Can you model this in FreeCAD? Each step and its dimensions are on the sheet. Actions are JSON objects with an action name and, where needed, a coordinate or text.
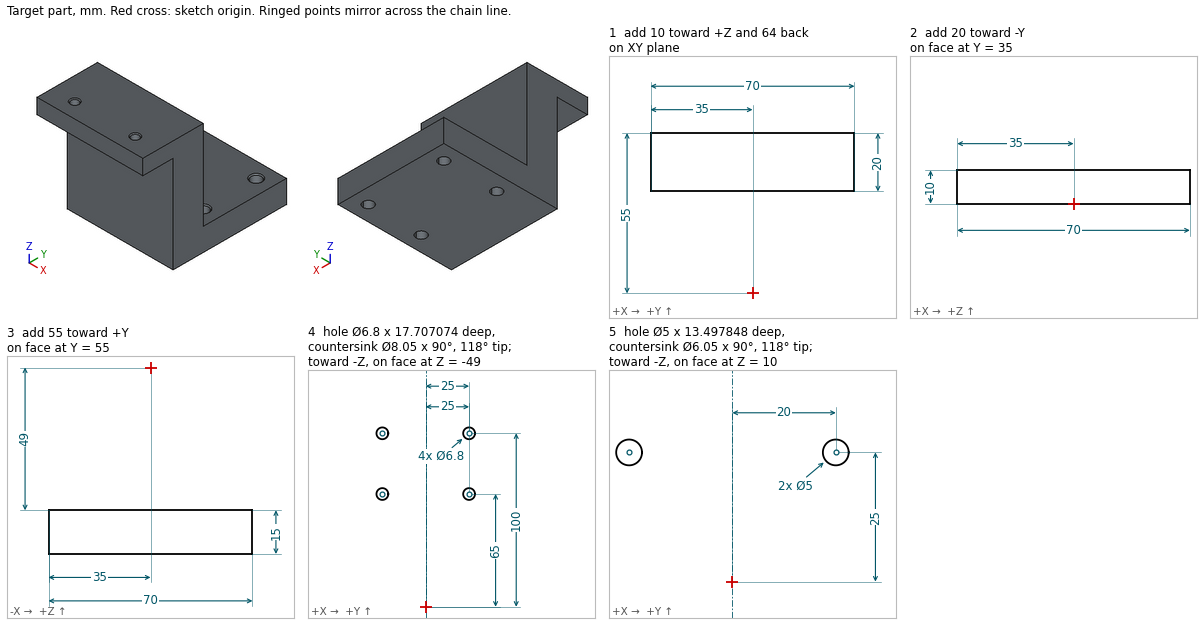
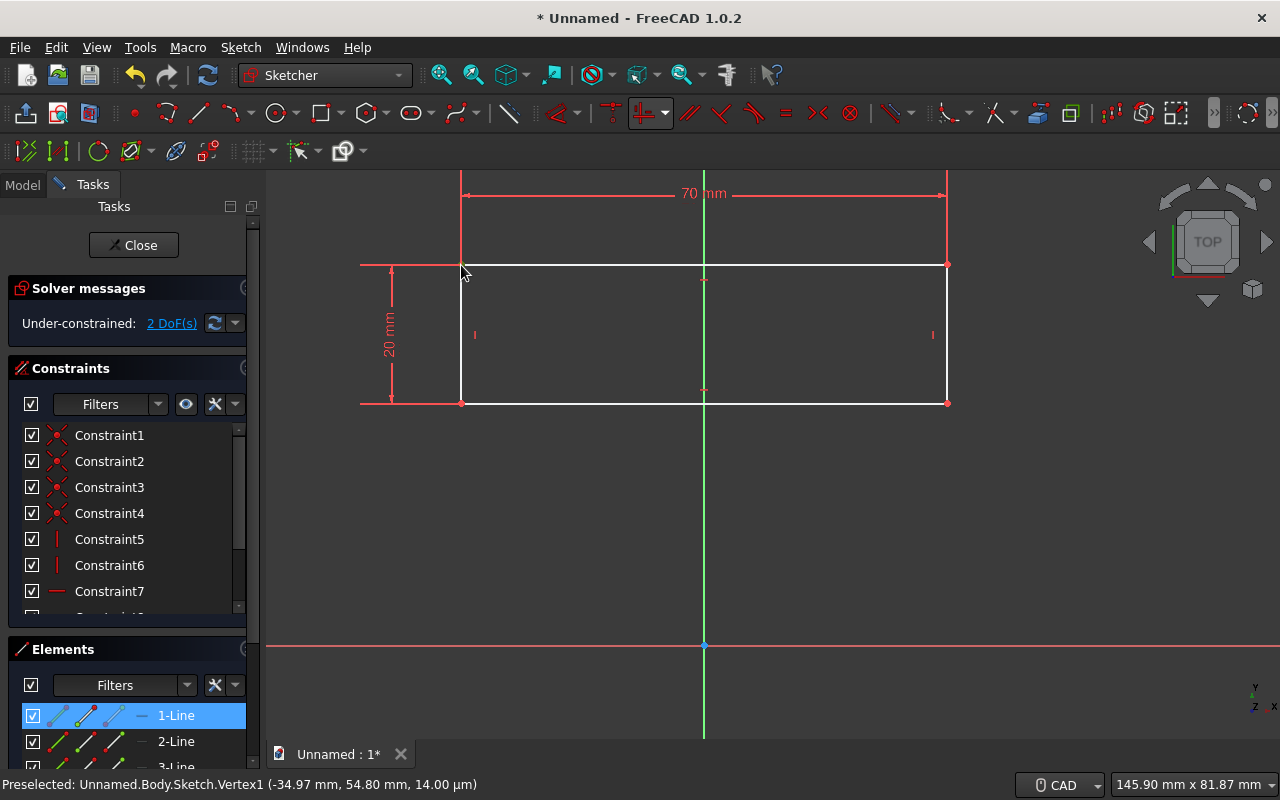
{"action": "left_click", "coordinate": [580, 114]}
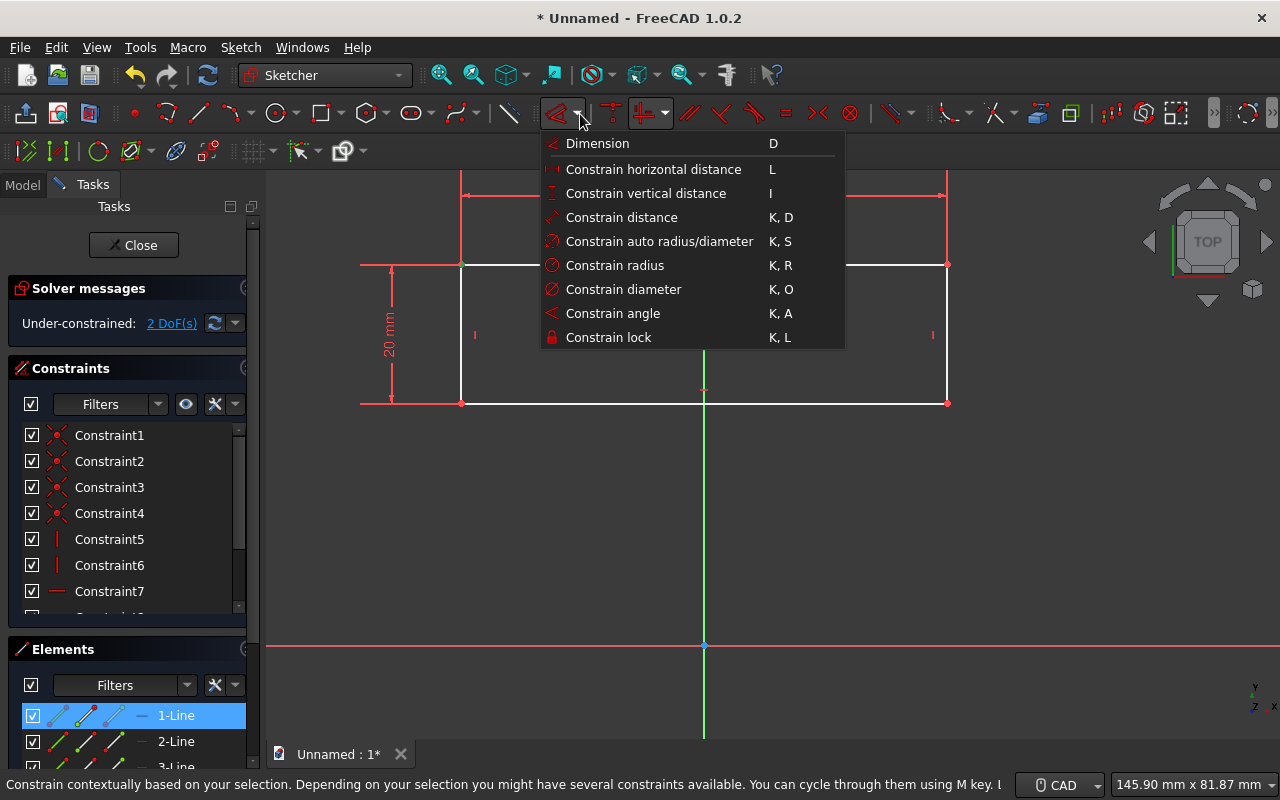
{"action": "left_click", "coordinate": [693, 169]}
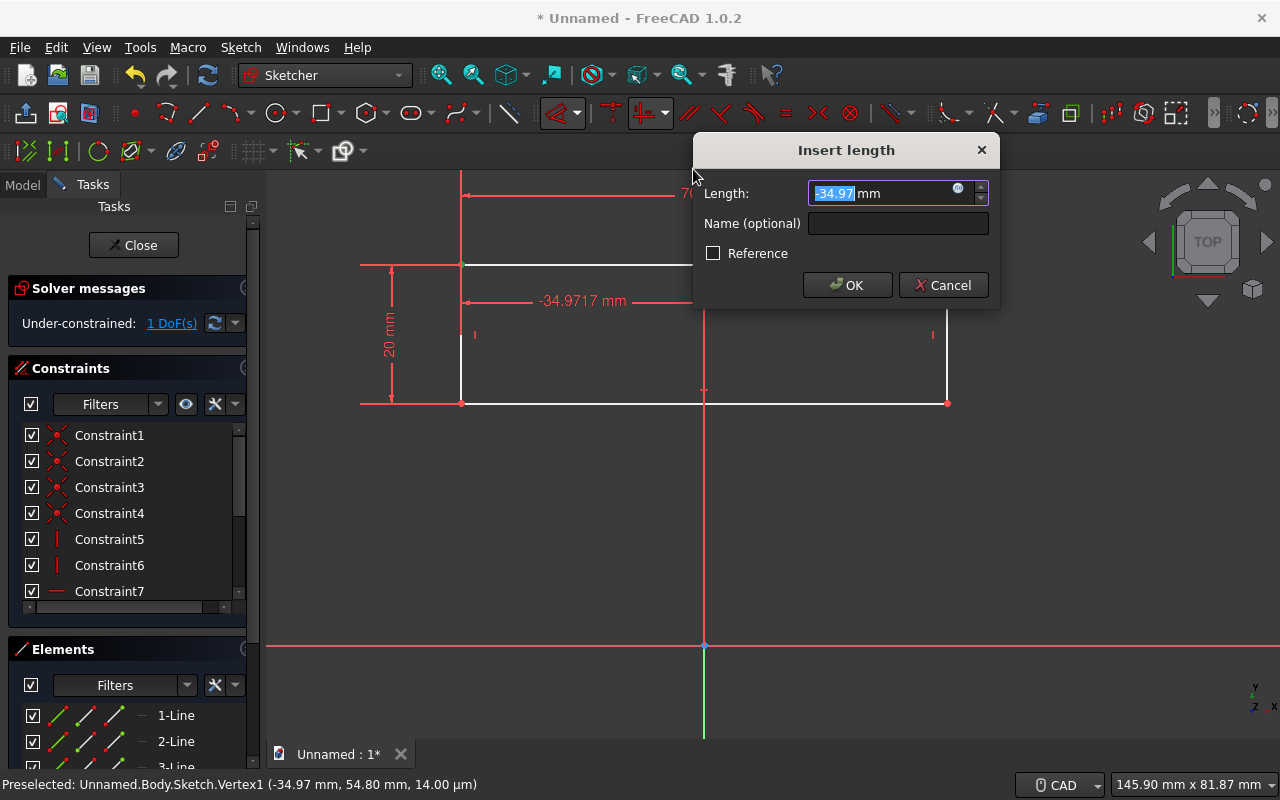
{"action": "type", "text": "-35"}
{"action": "key", "text": "Return"}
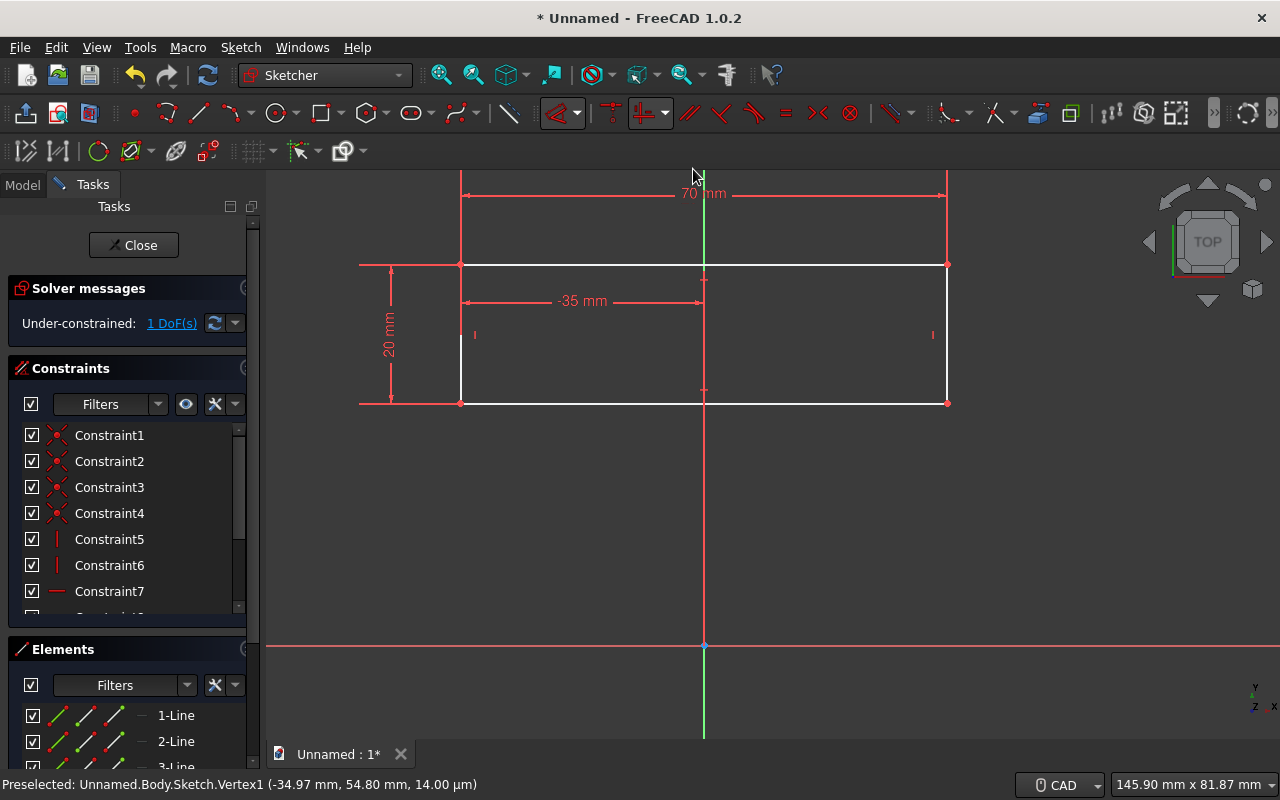
{"action": "left_click", "coordinate": [461, 265]}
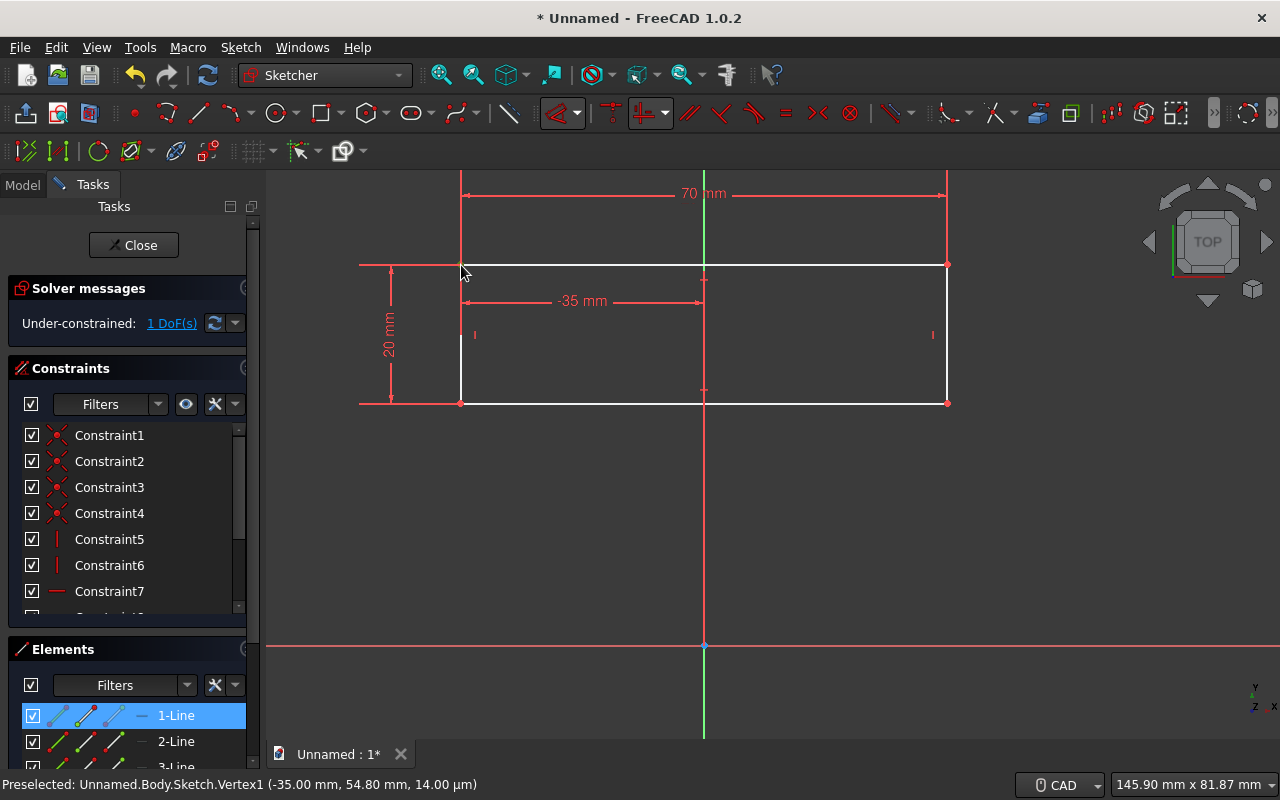
{"action": "left_click", "coordinate": [580, 114]}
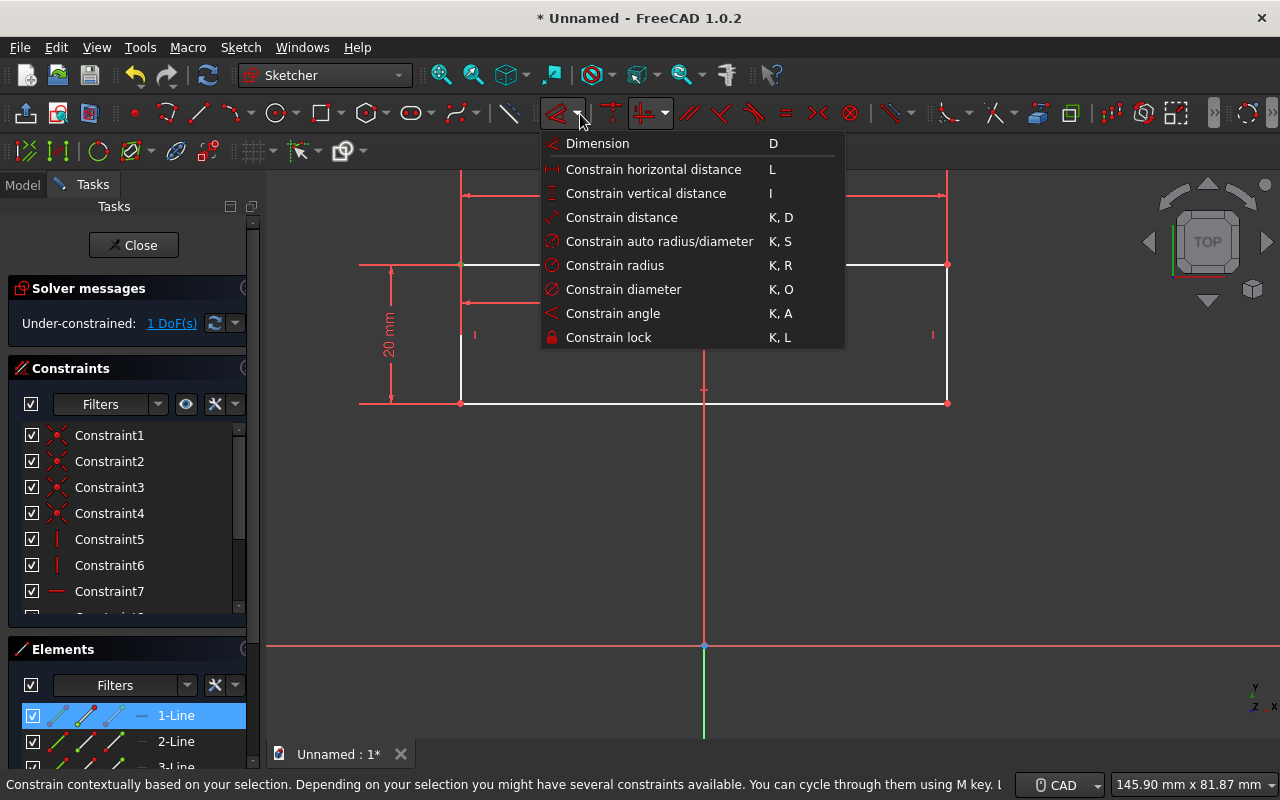
{"action": "left_click", "coordinate": [693, 193]}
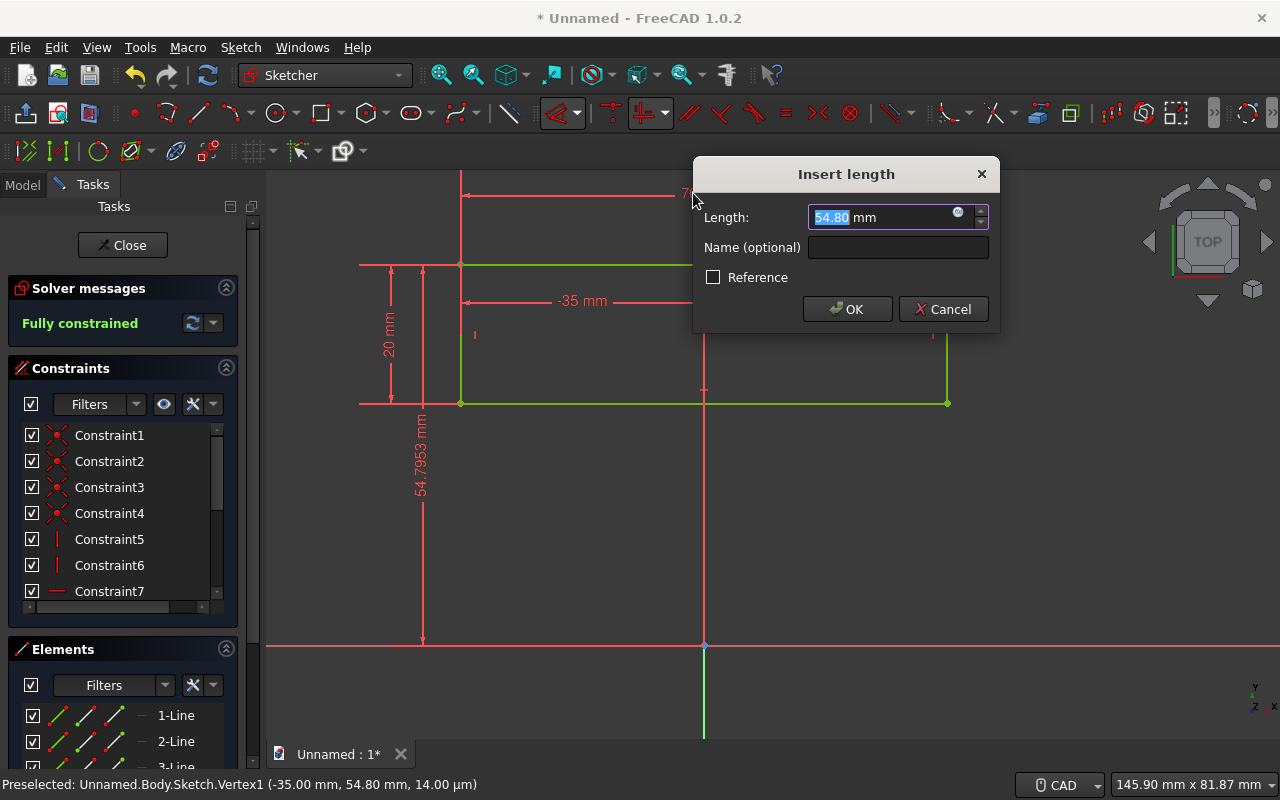
{"action": "type", "text": "55"}
{"action": "key", "text": "Return"}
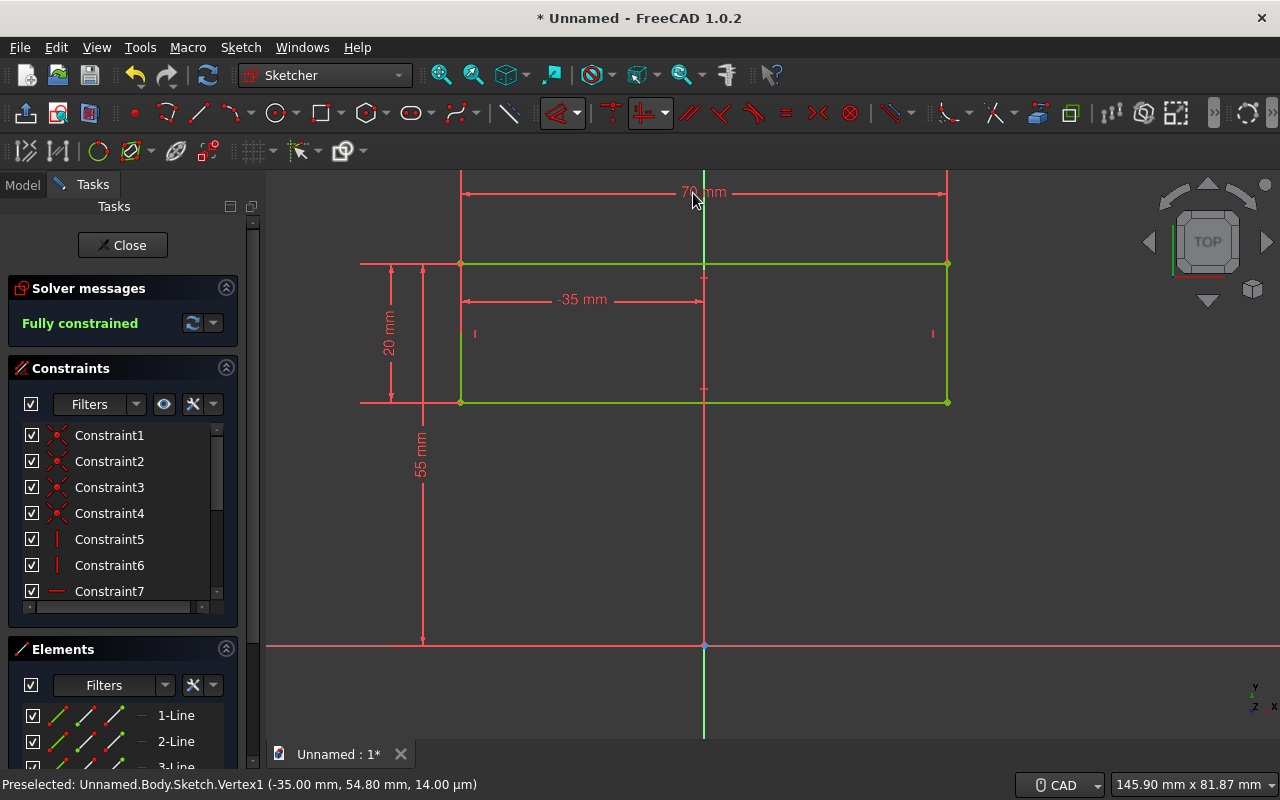
{"action": "left_click", "coordinate": [123, 245]}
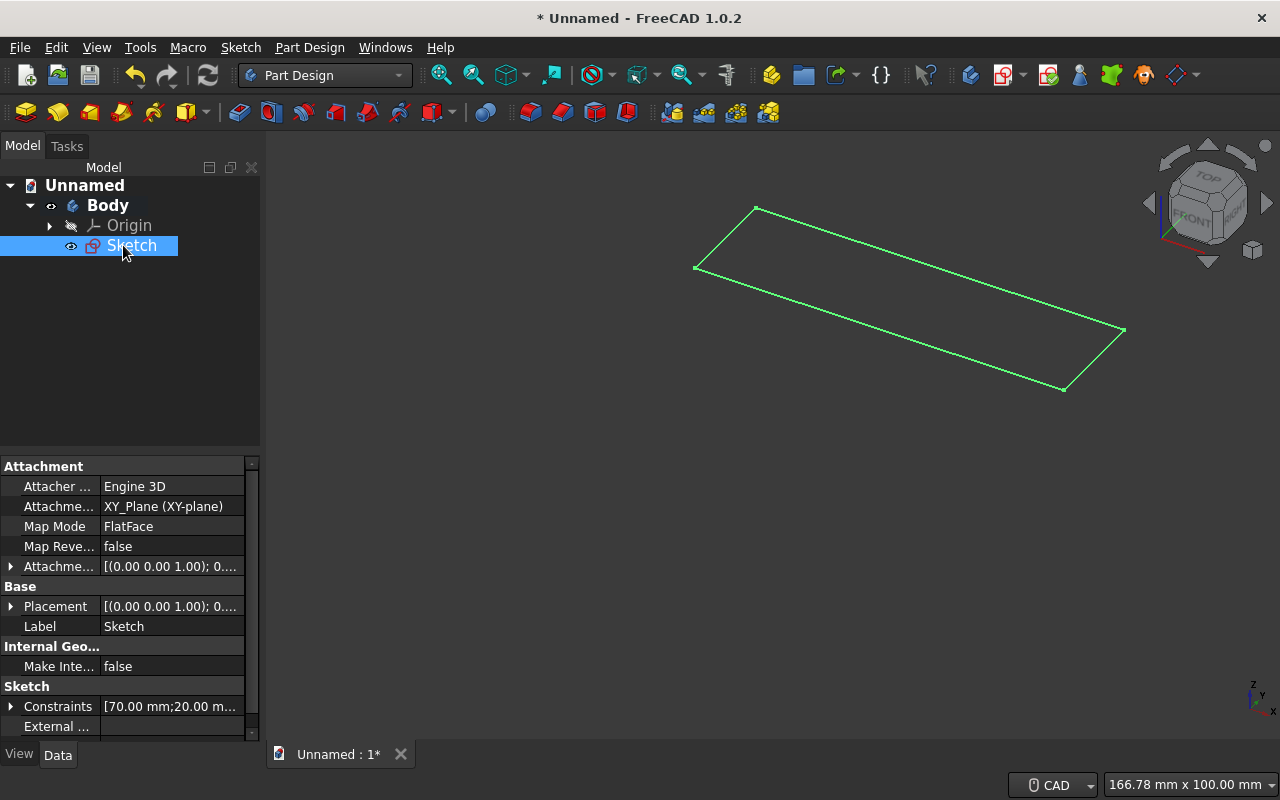
{"action": "left_click", "coordinate": [26, 112]}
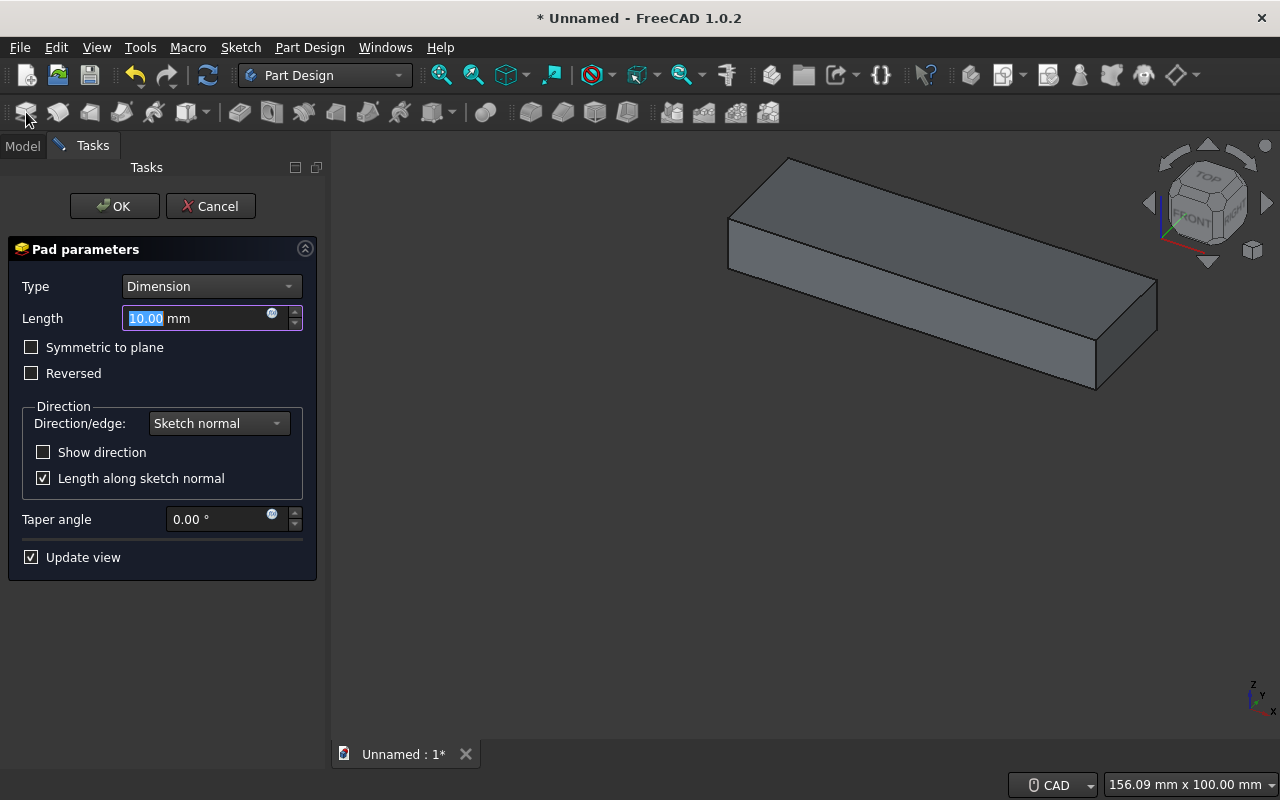
{"action": "left_click", "coordinate": [212, 286]}